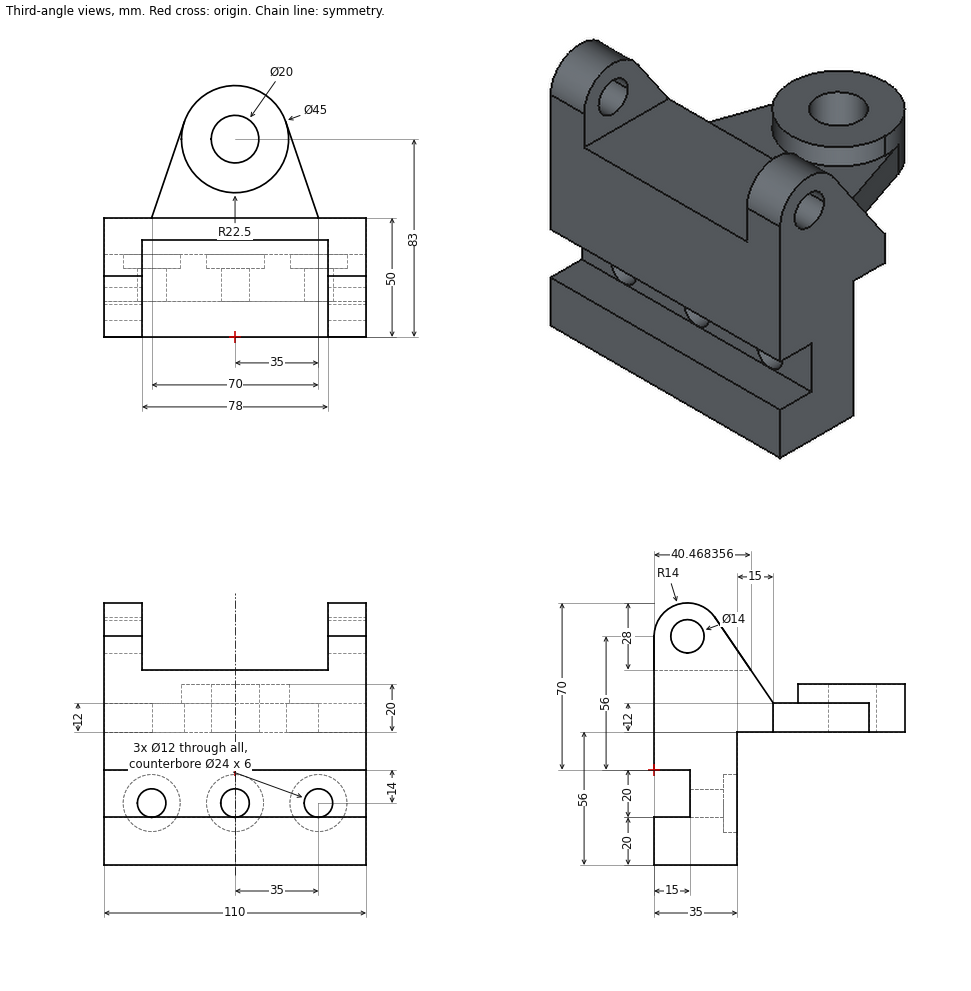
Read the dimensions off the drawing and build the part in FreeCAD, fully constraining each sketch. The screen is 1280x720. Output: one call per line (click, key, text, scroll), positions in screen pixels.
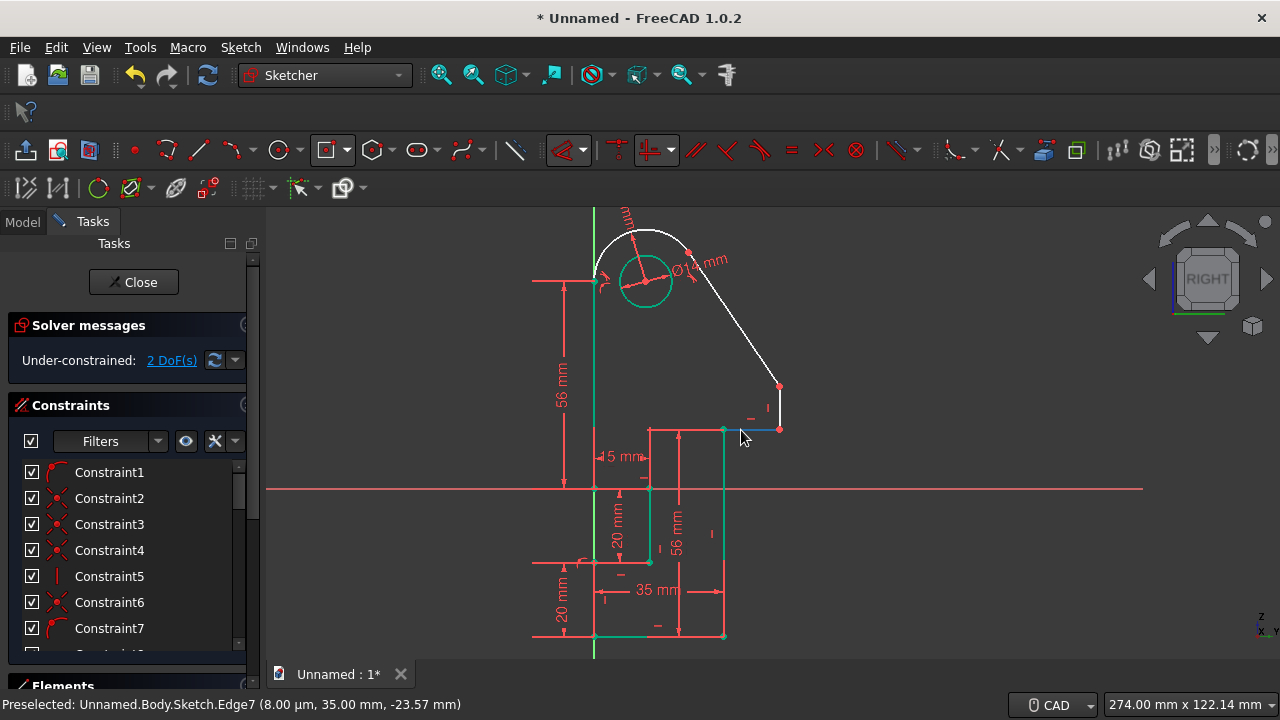
click(740, 430)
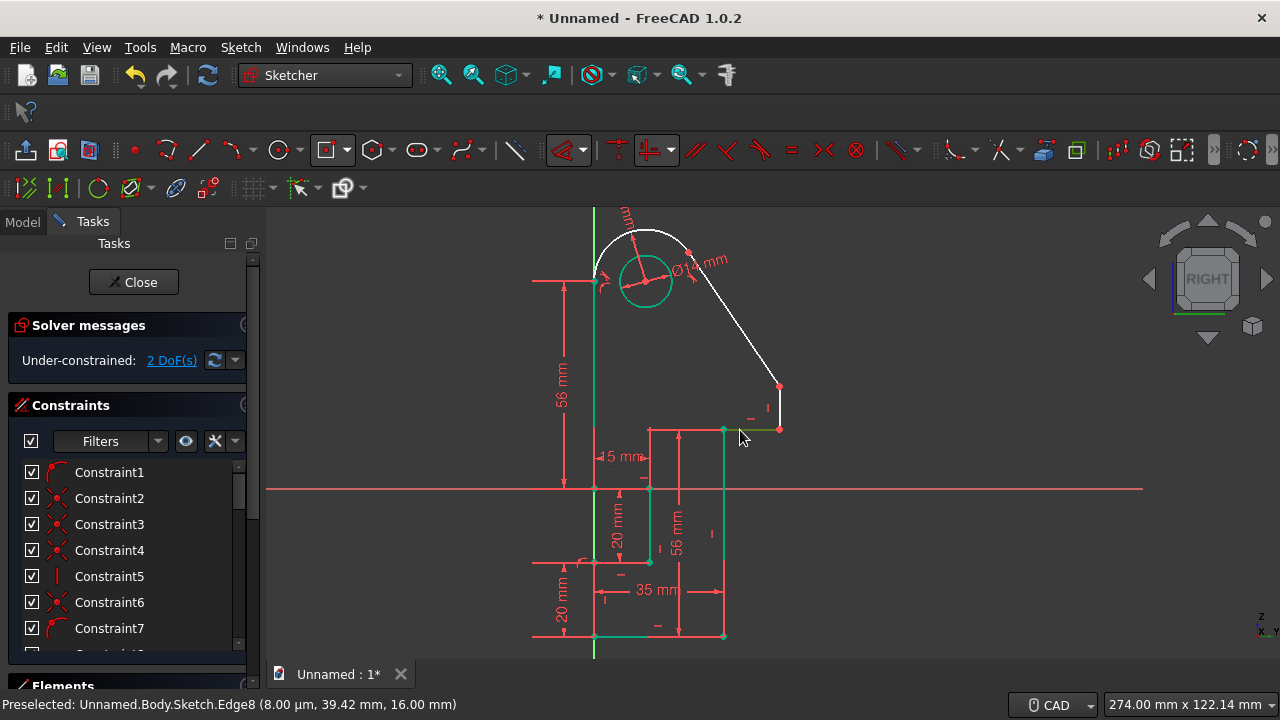
click(586, 150)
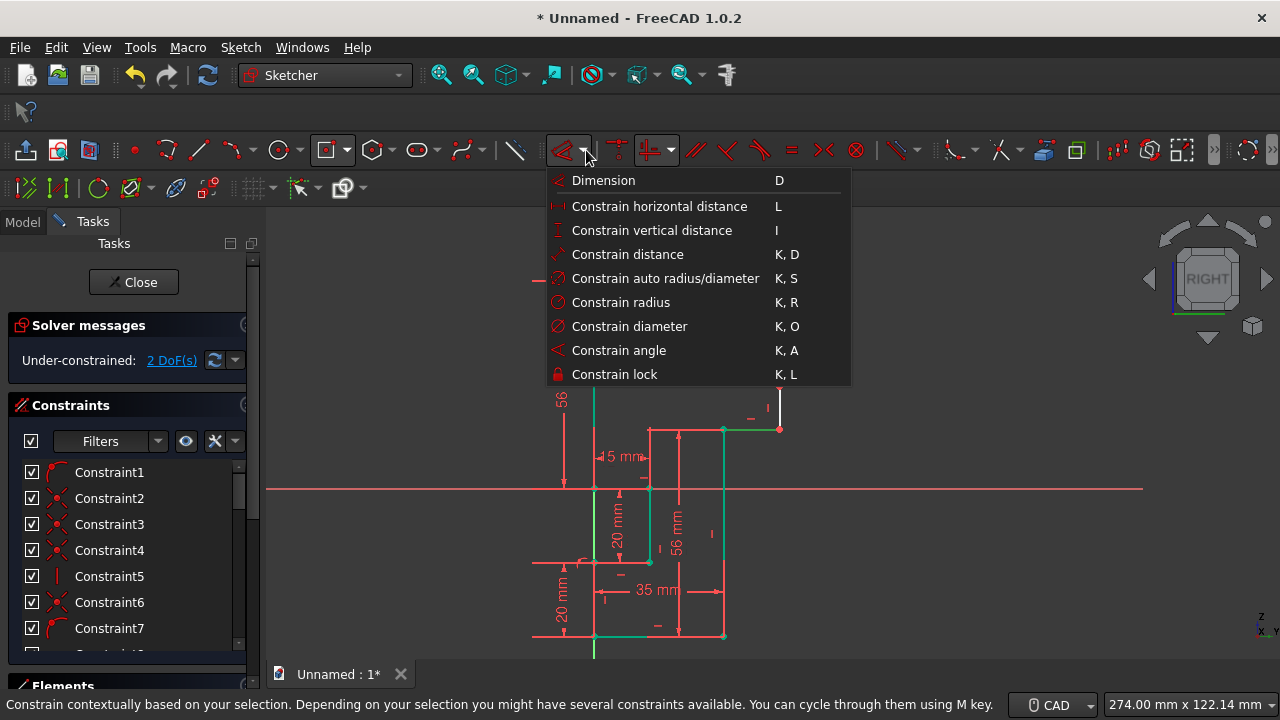
click(699, 206)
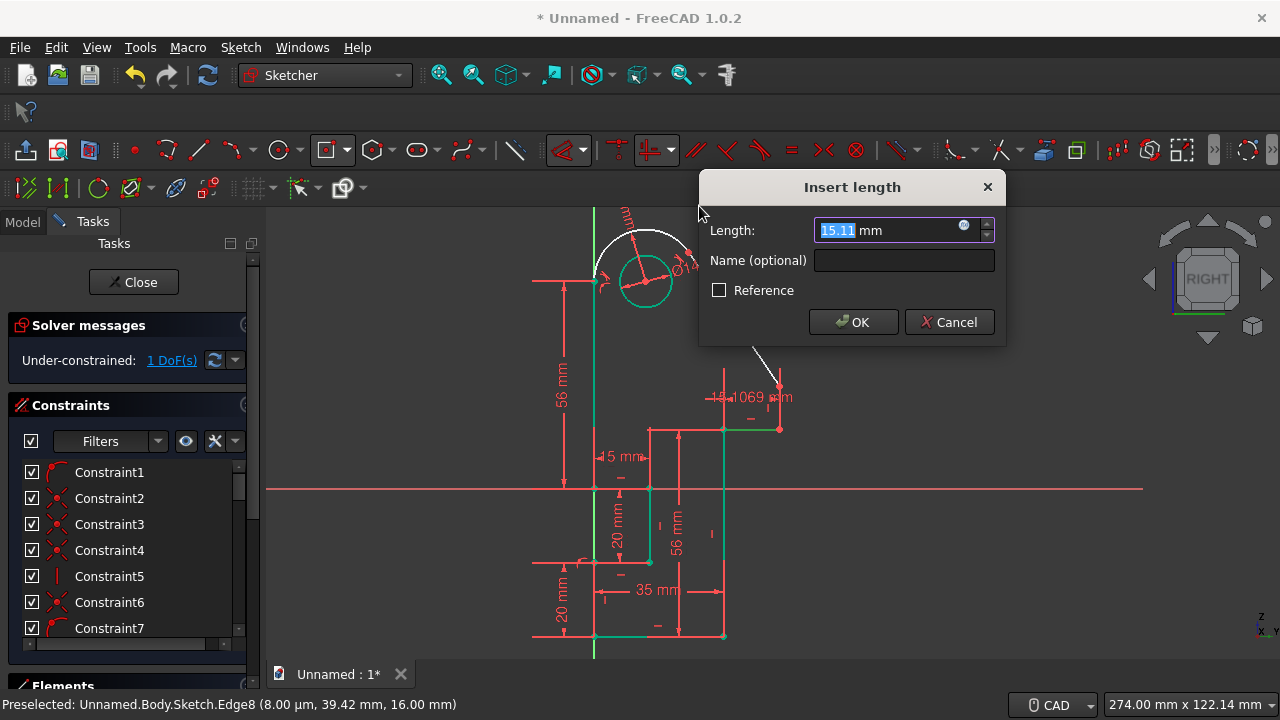
text(15)
key(Return)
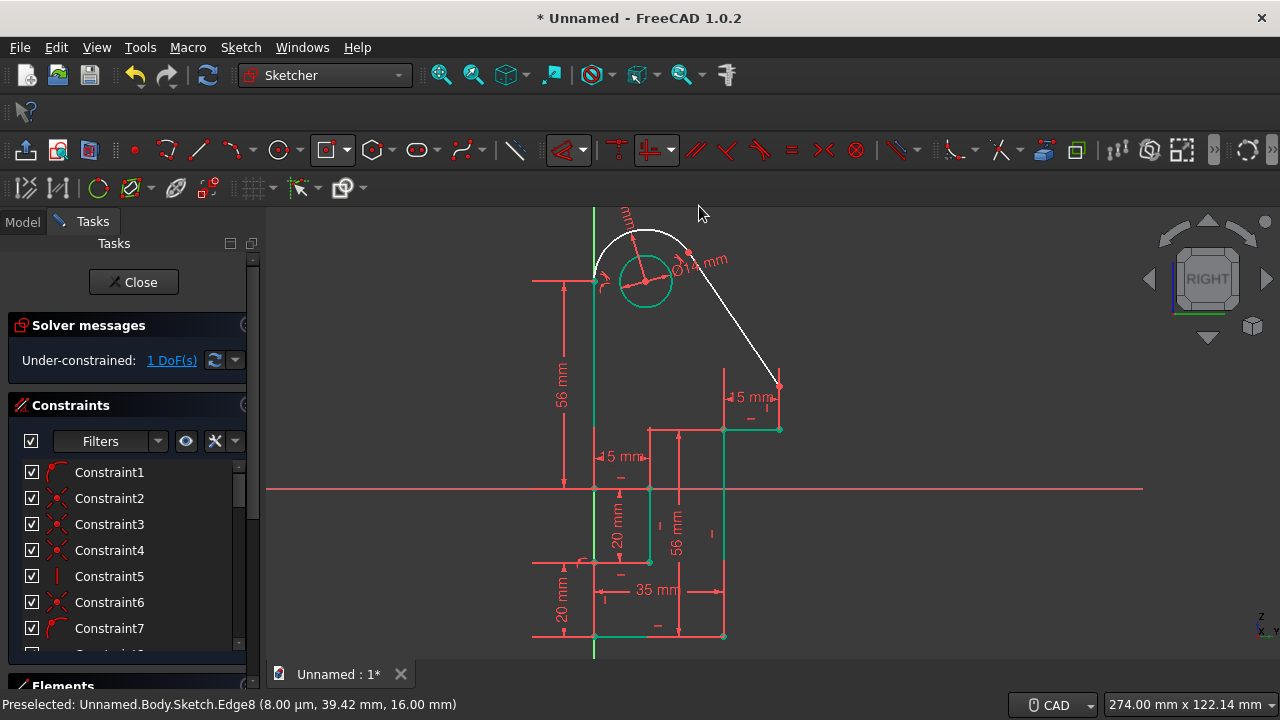
click(779, 416)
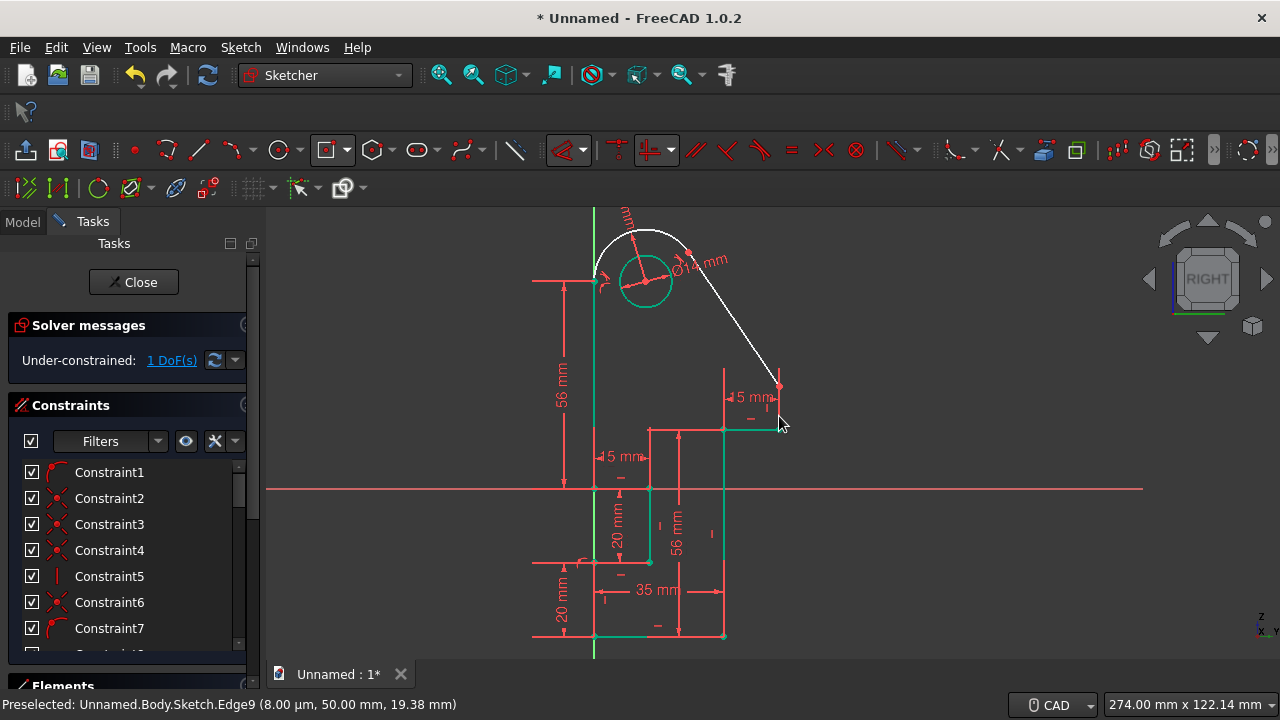
key(i)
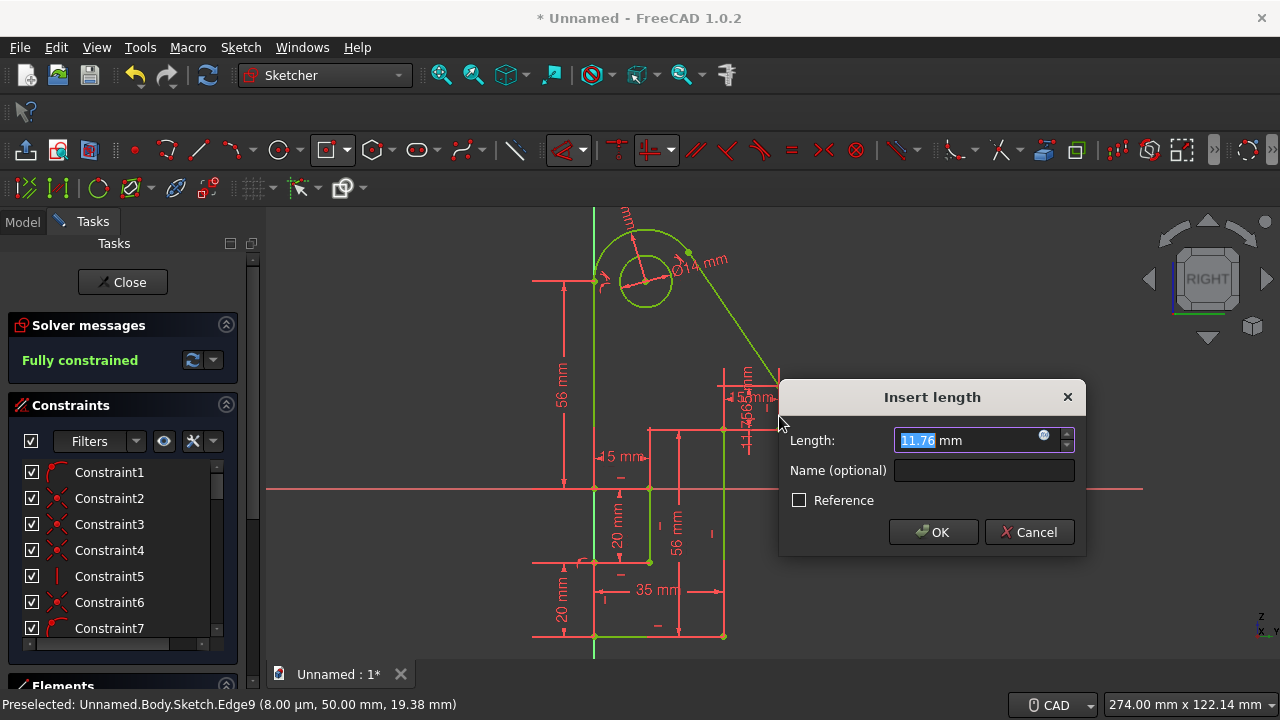
text(12)
key(Return)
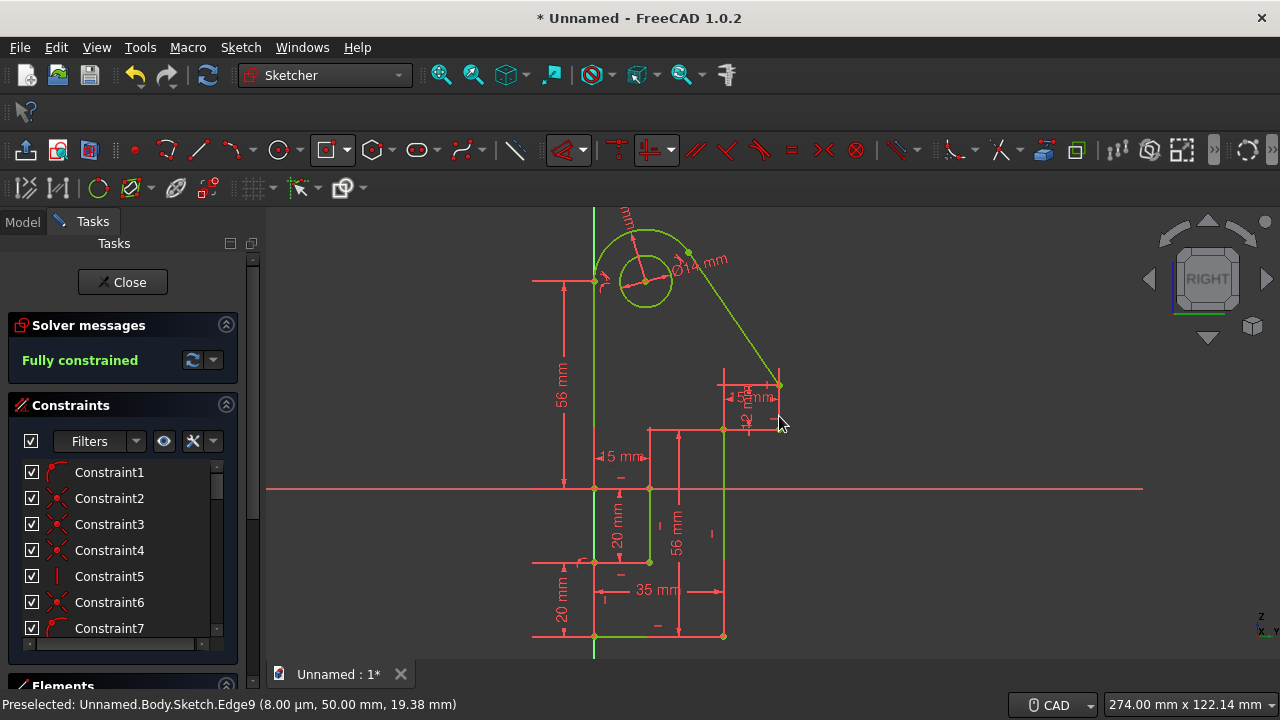
click(123, 282)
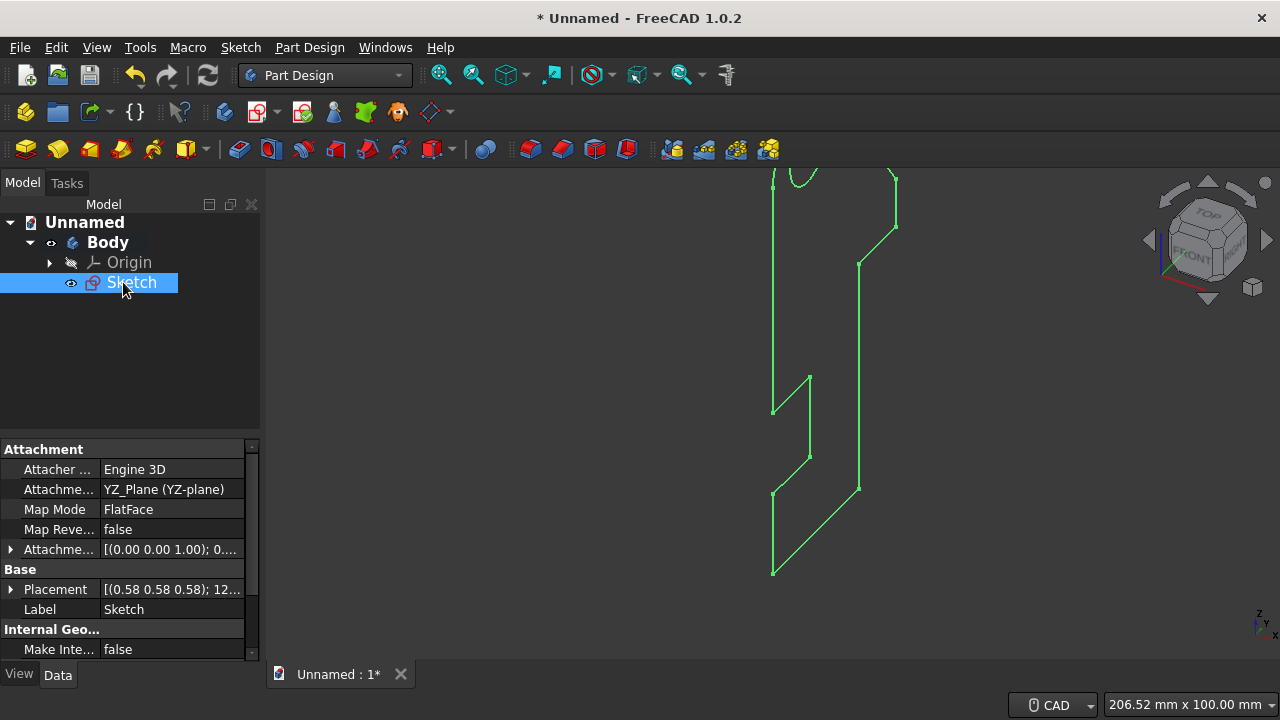
click(26, 150)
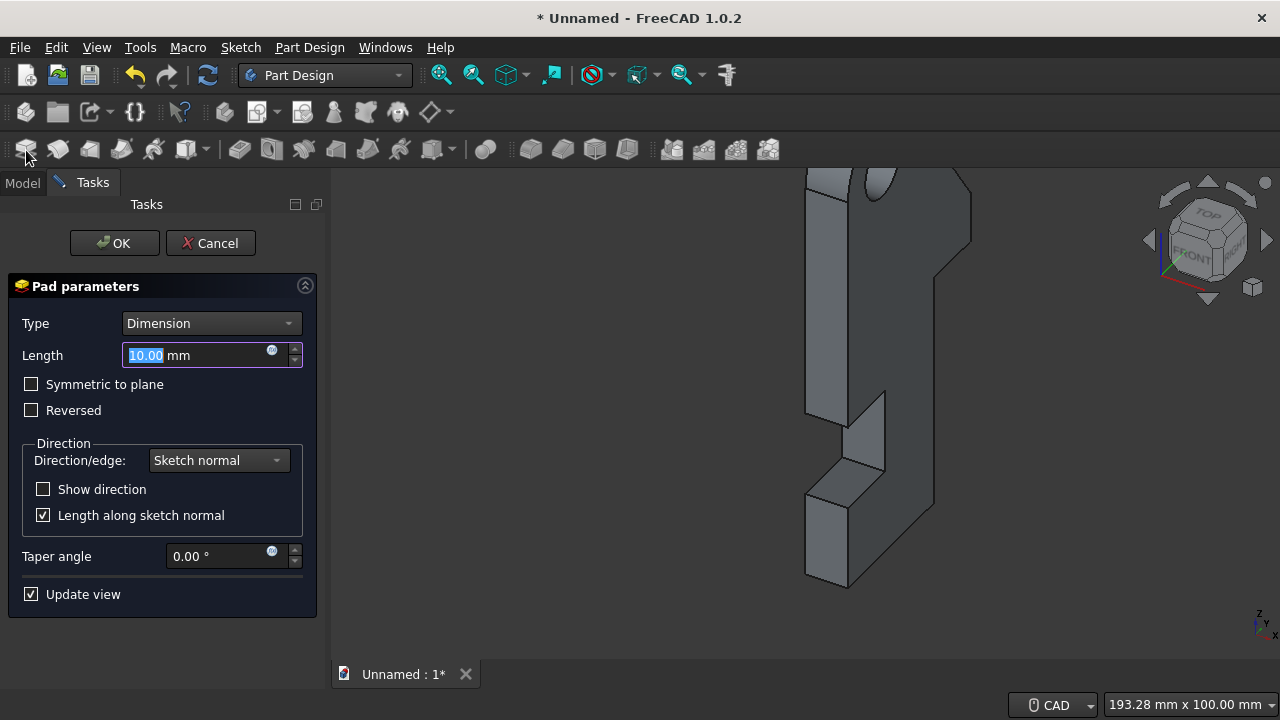
text(110)
key(Tab)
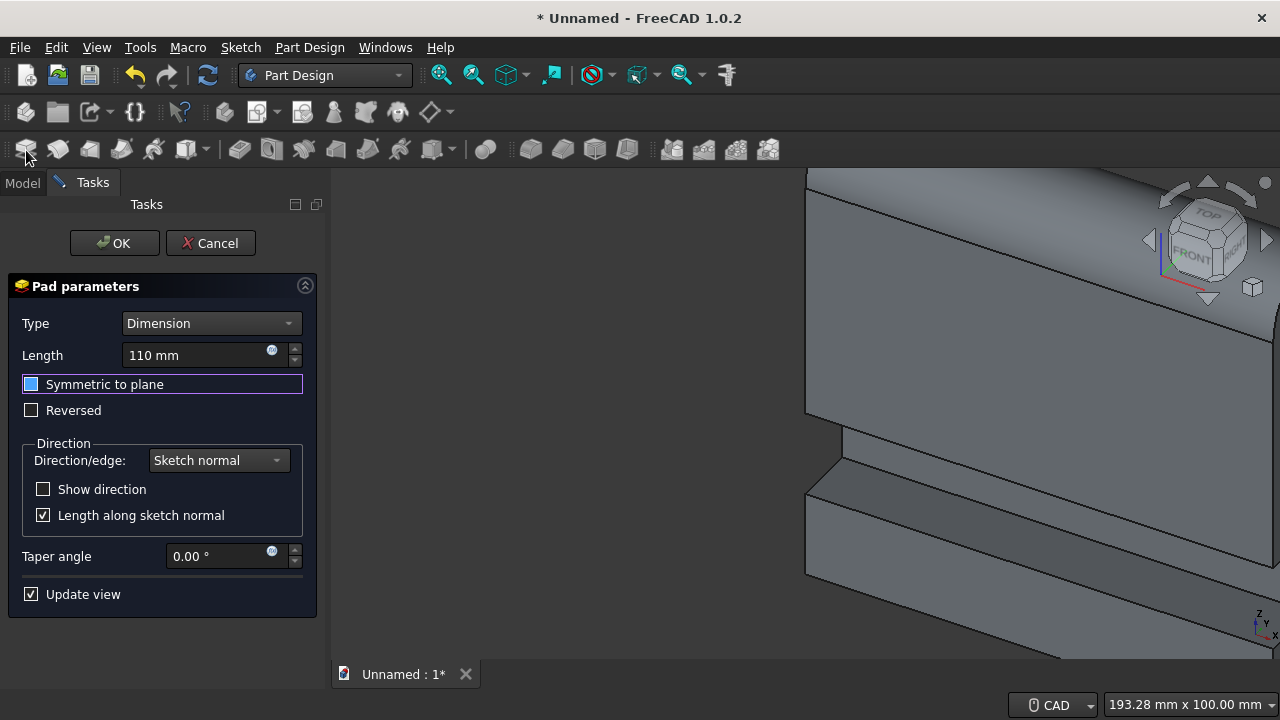
click(30, 384)